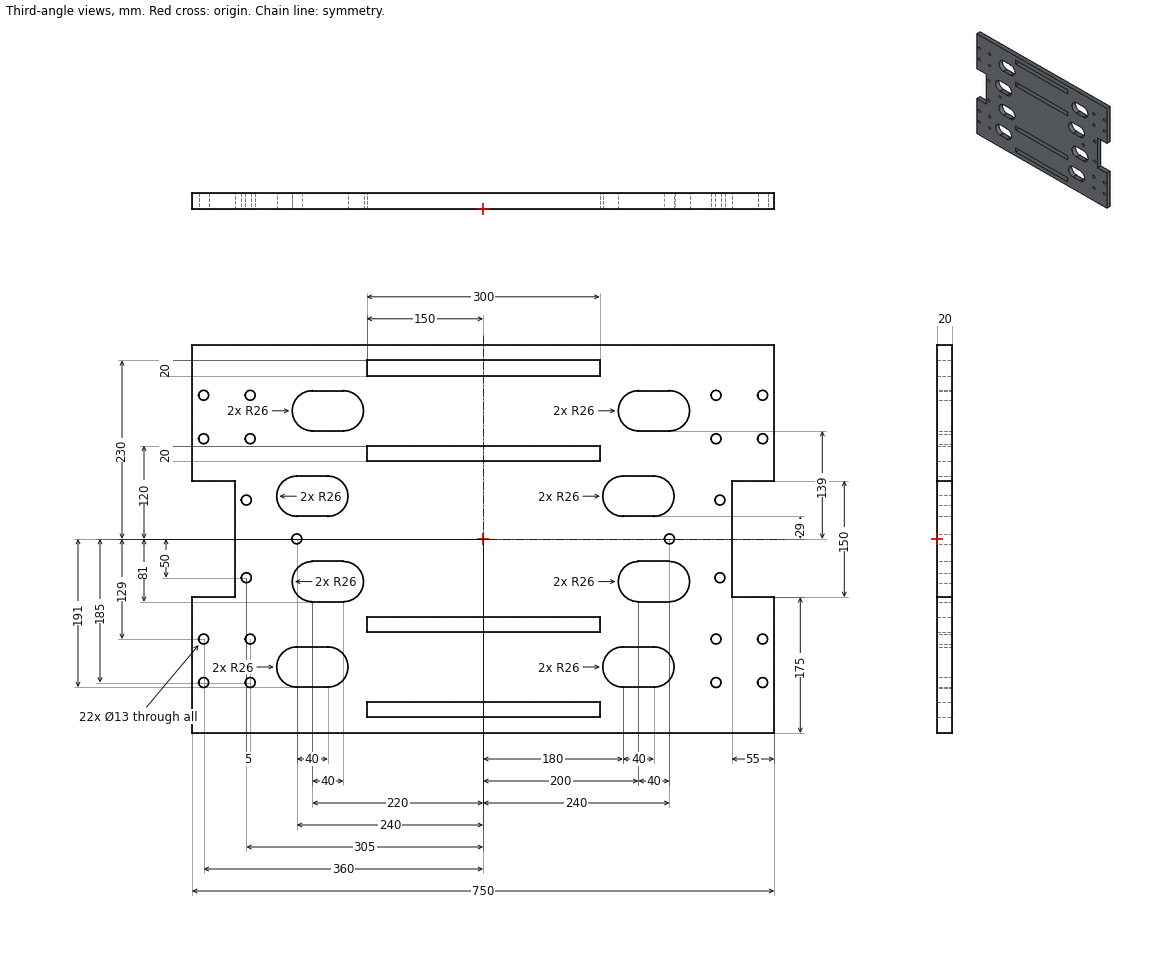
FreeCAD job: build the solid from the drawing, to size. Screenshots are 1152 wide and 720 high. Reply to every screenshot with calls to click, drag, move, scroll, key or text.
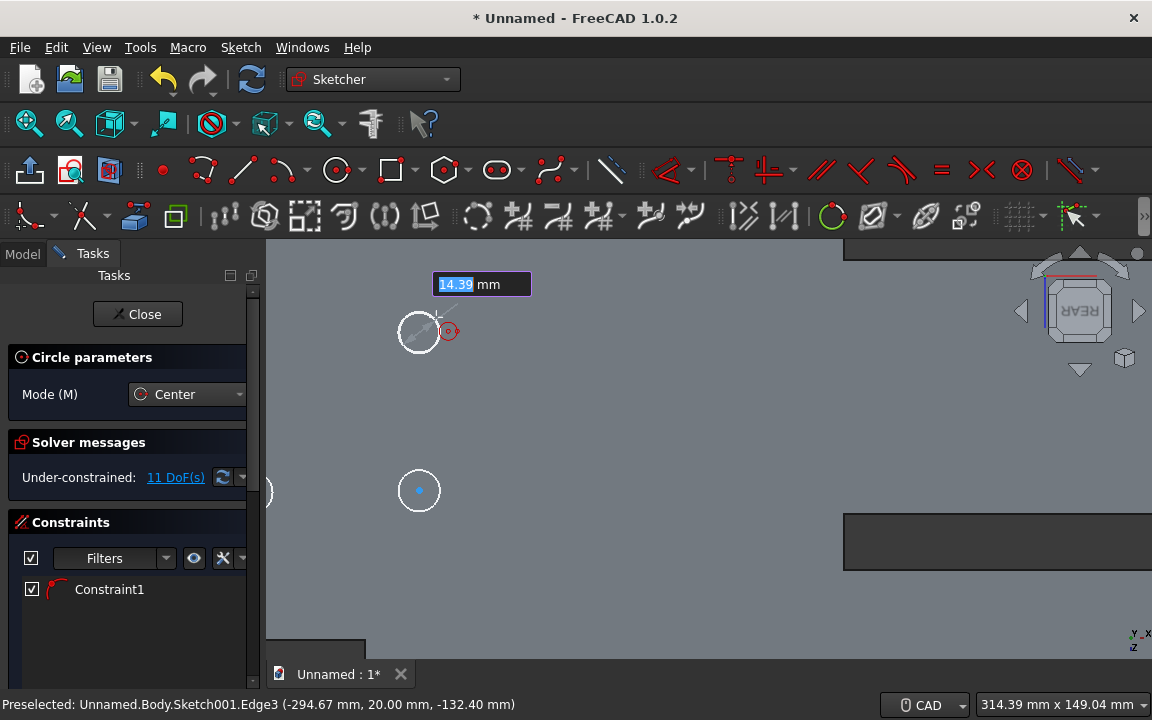
click(434, 317)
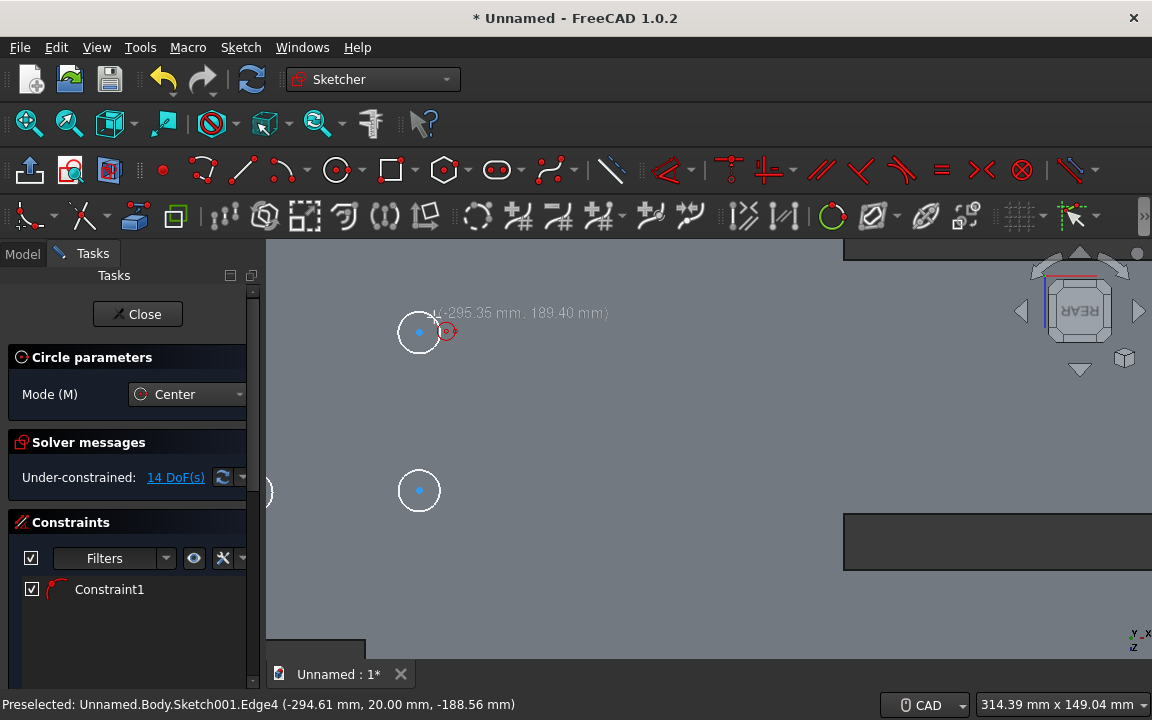
scroll(436, 317, down, 7)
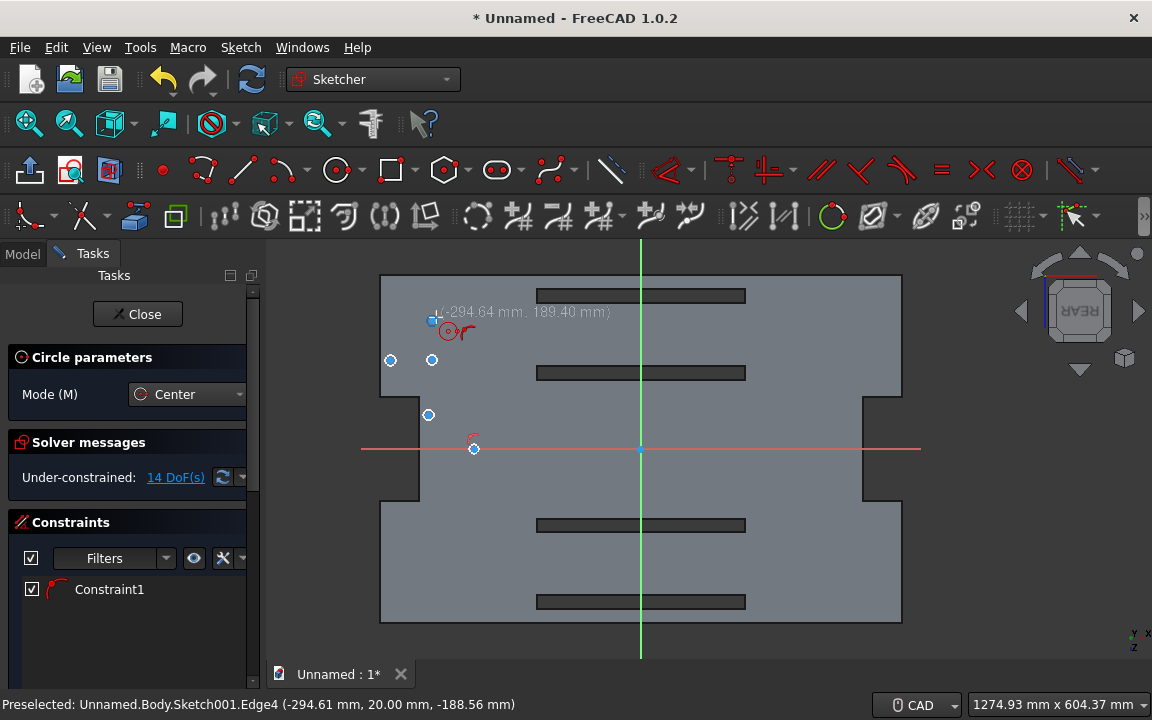
scroll(391, 320, up, 9)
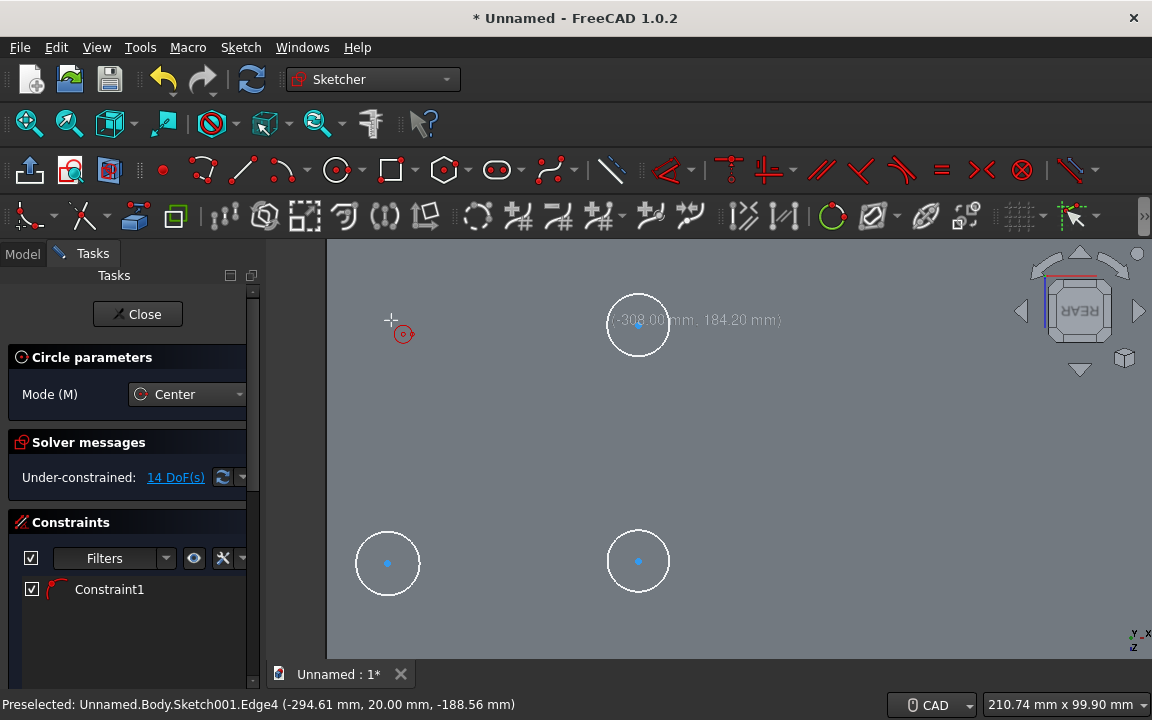
scroll(391, 320, down, 9)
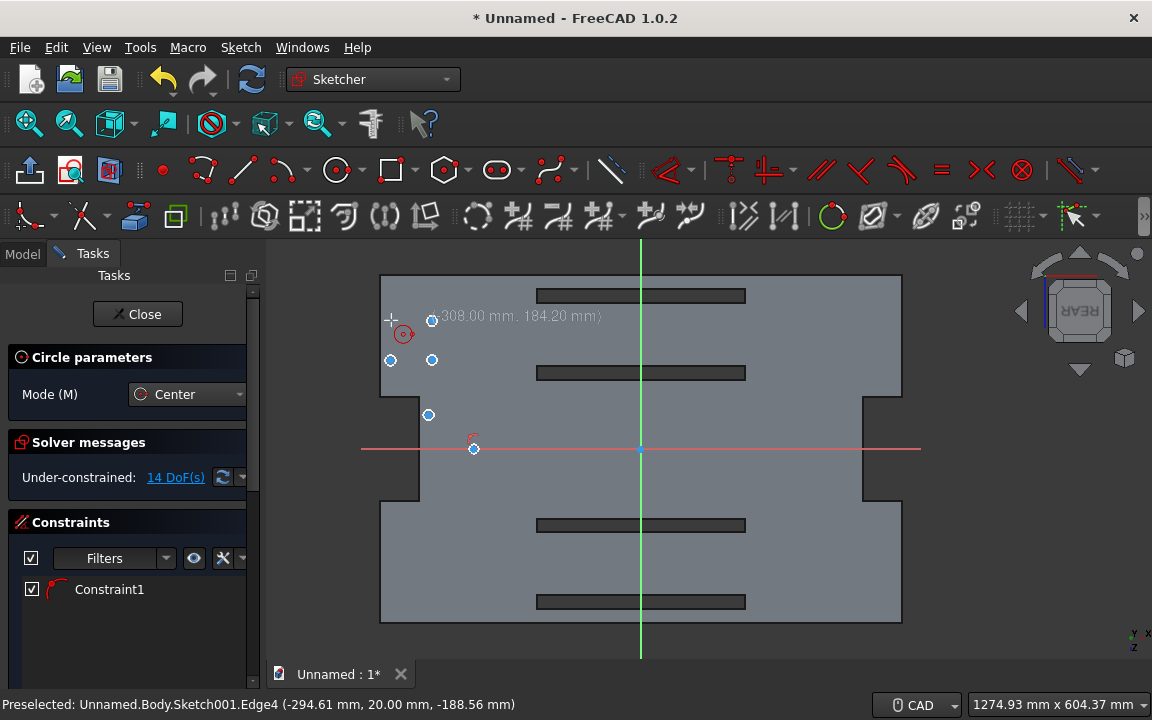
click(391, 320)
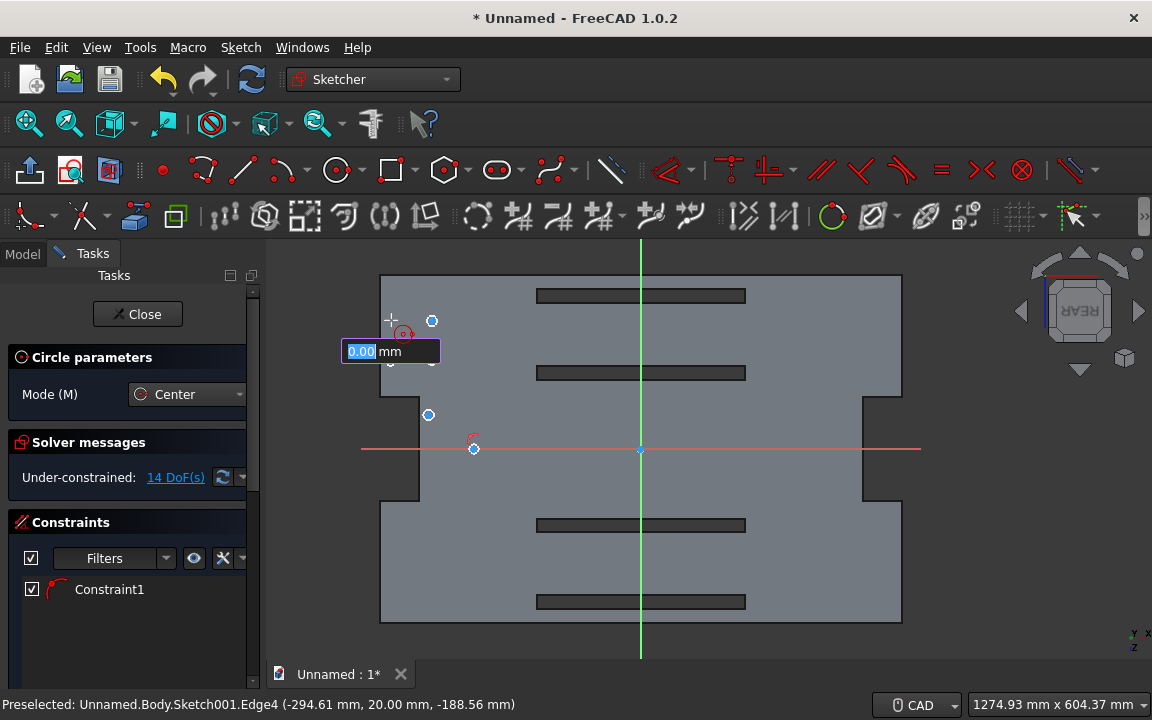
scroll(394, 317, up, 7)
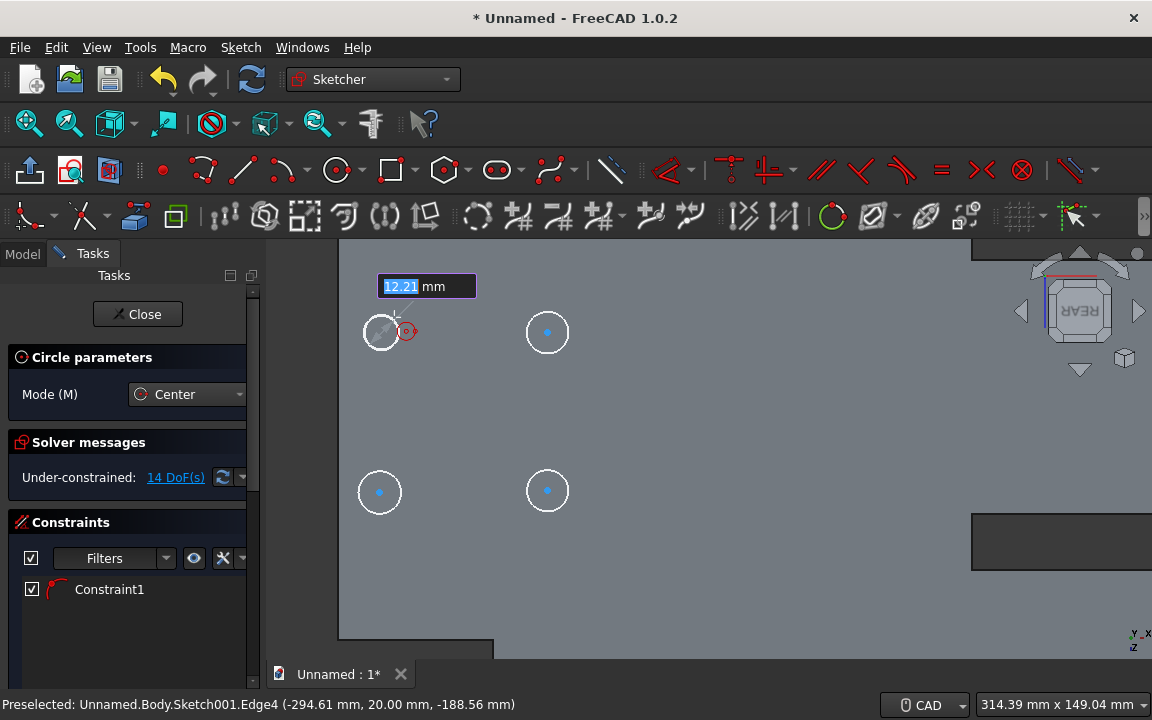
click(393, 317)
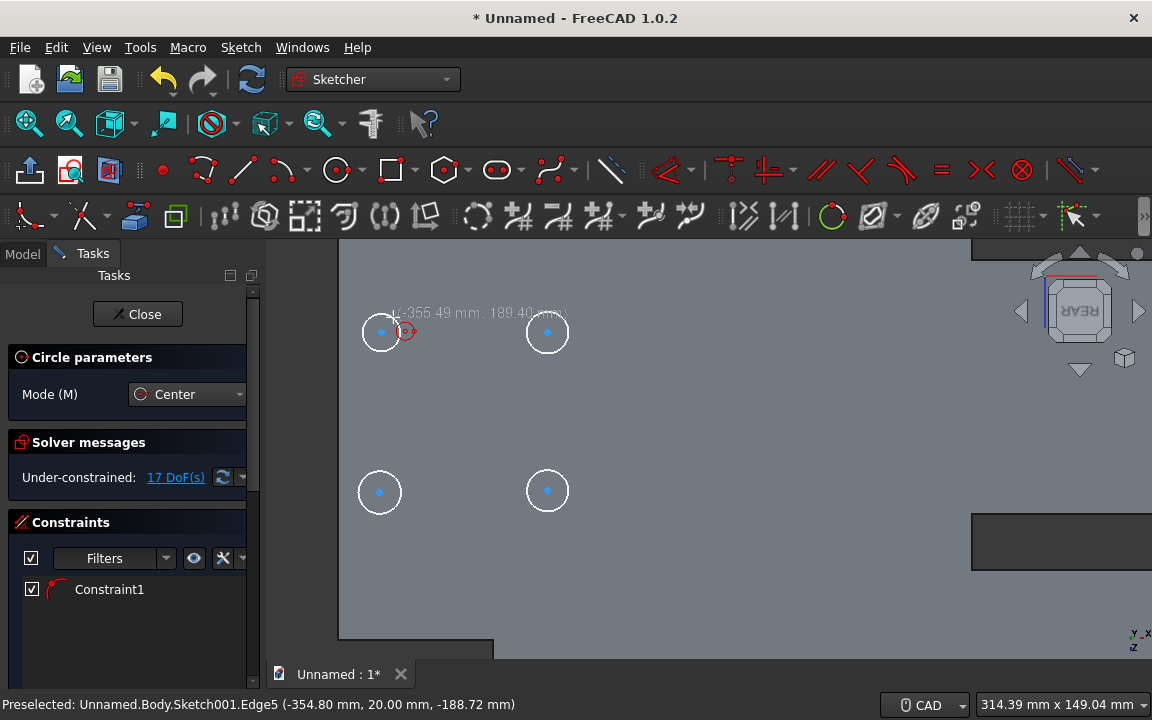
scroll(394, 317, down, 7)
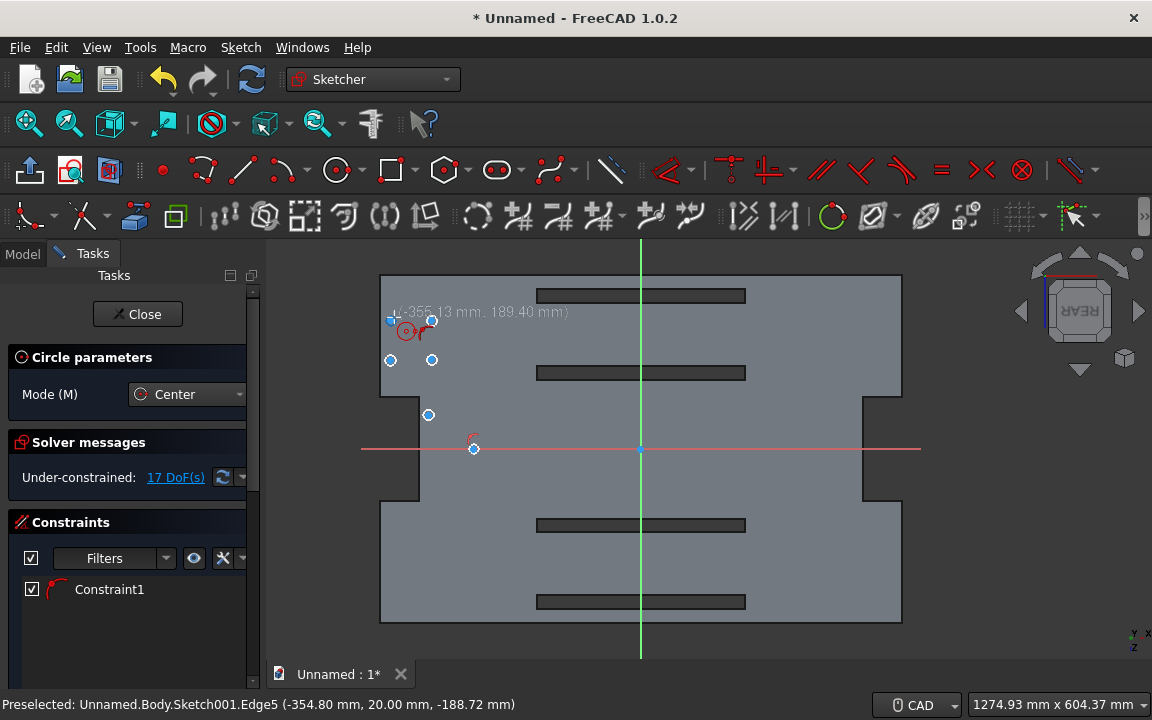
scroll(391, 539, up, 9)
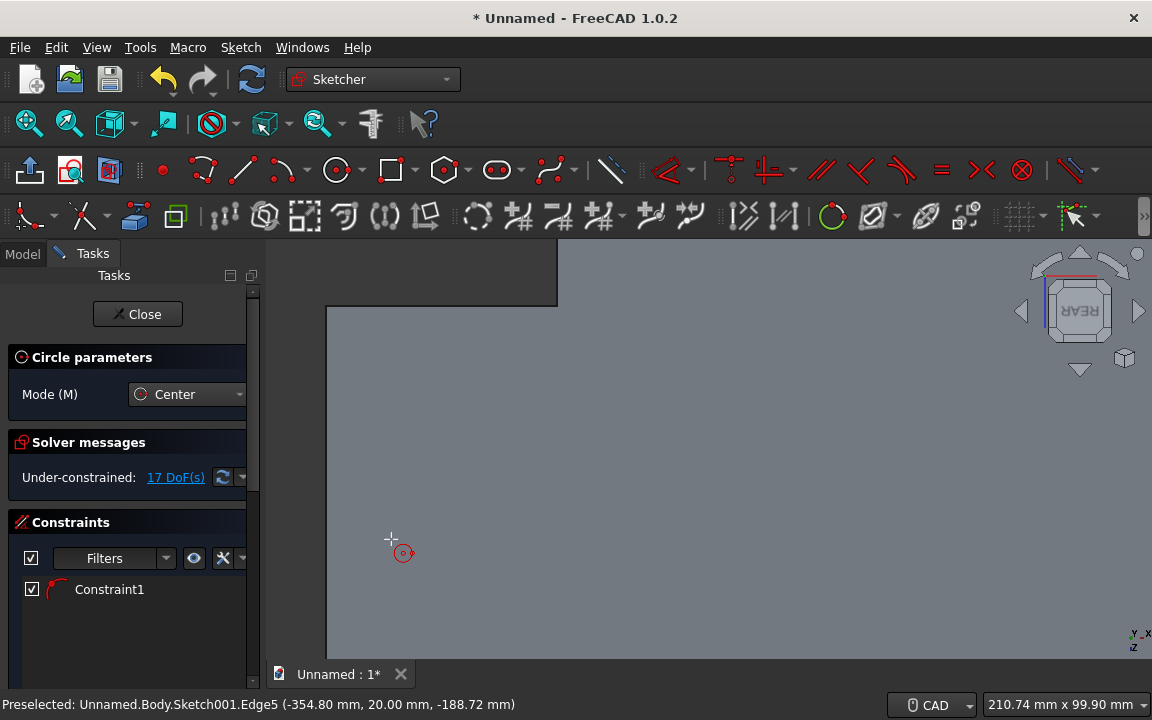
scroll(391, 540, down, 9)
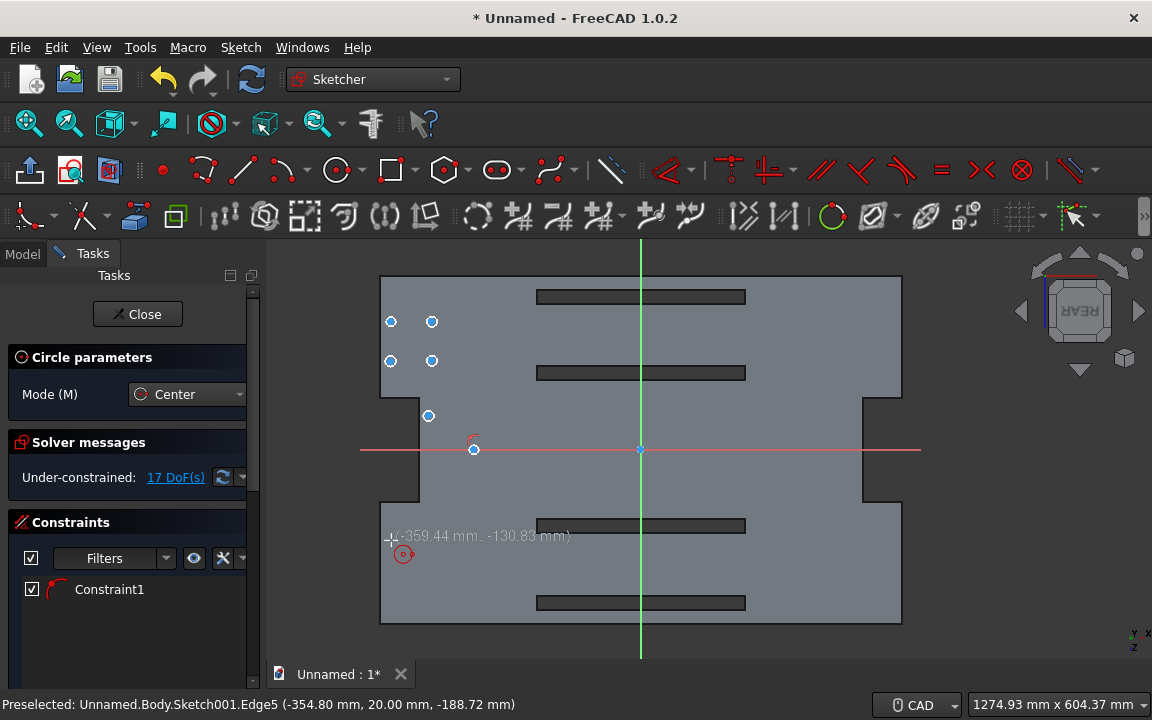
click(391, 539)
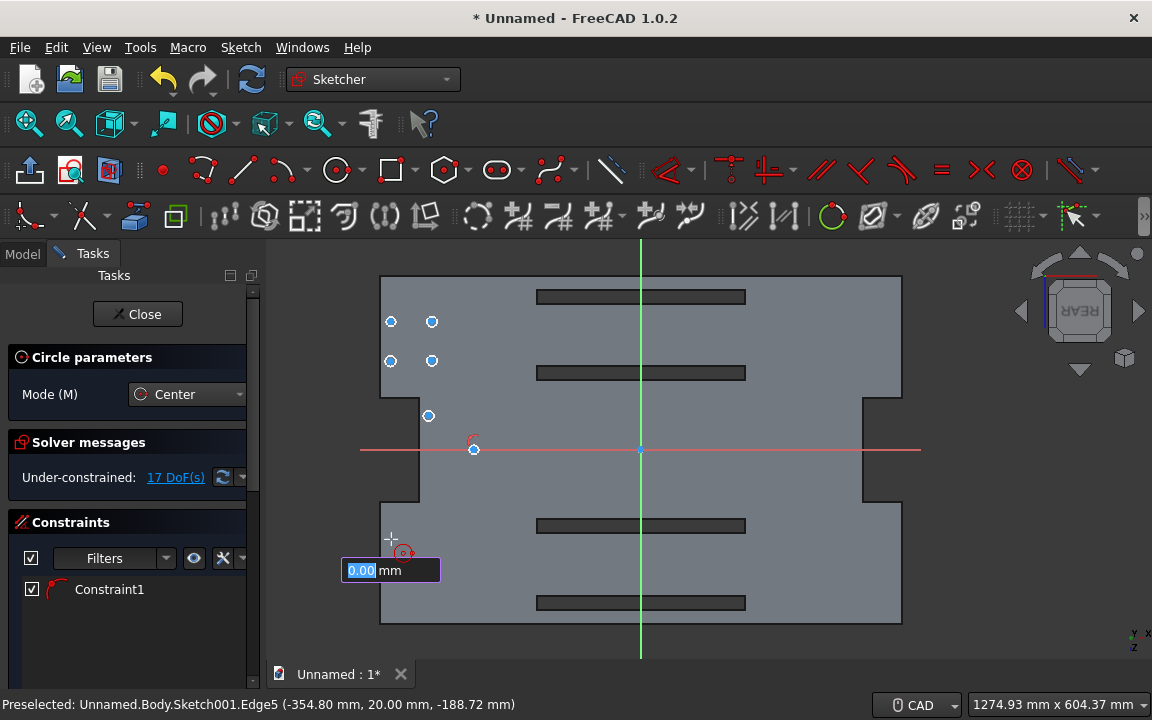
scroll(394, 536, up, 7)